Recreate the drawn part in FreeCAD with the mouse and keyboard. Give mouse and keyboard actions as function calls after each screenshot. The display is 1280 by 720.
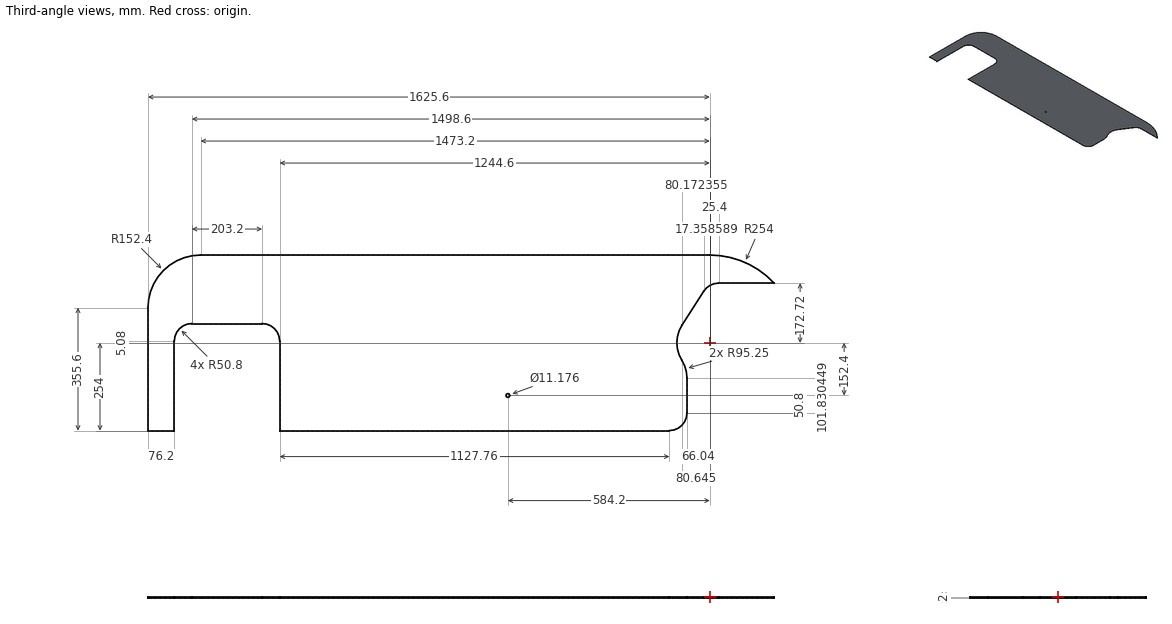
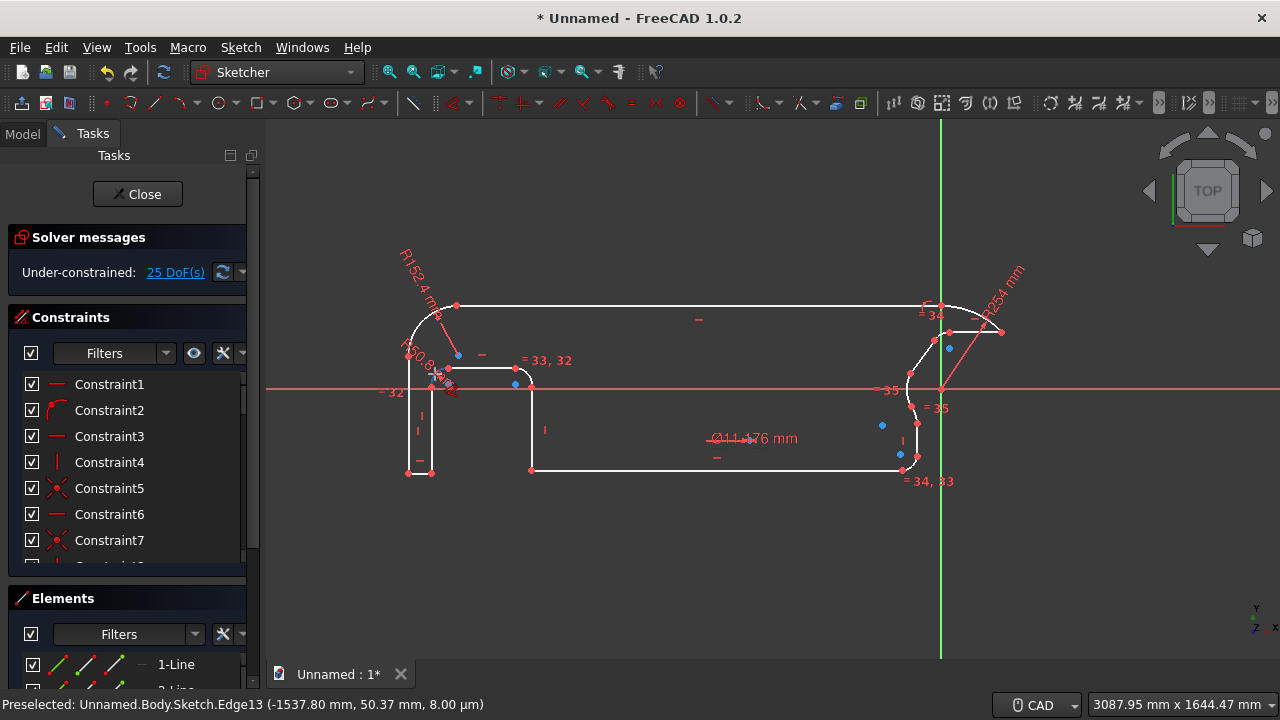
scroll(916, 418, up, 5)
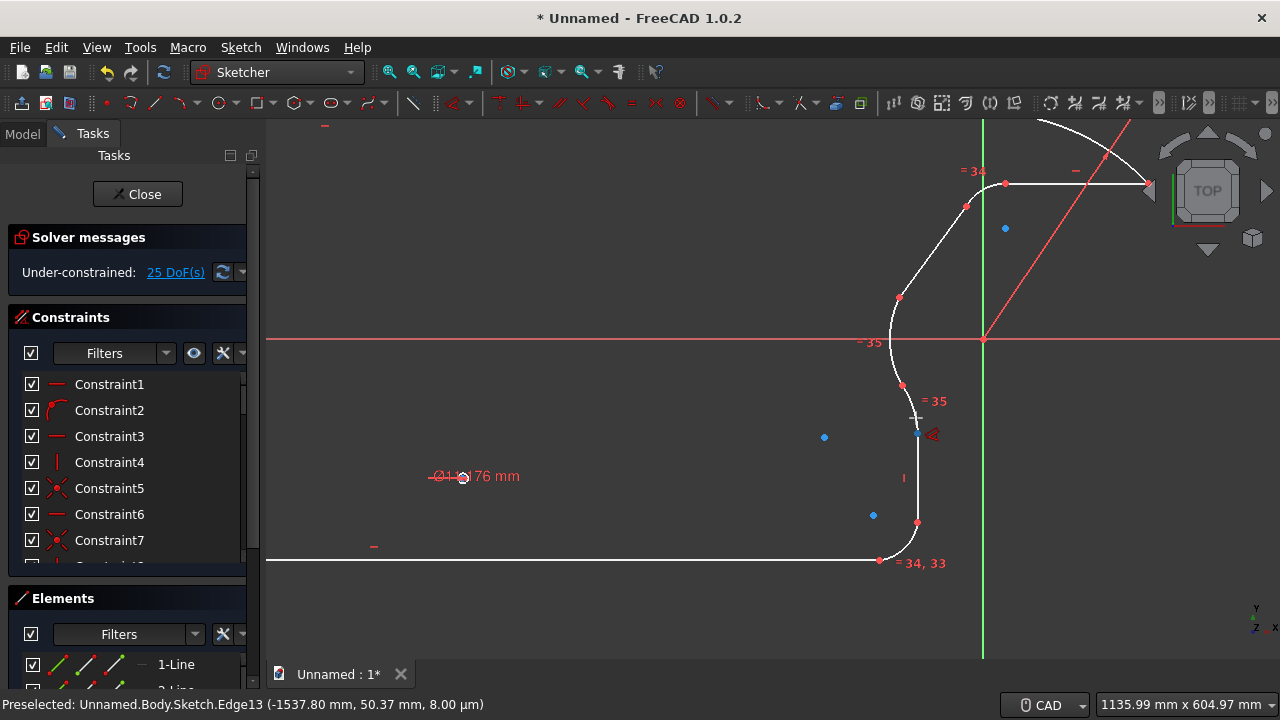
click(916, 418)
click(947, 411)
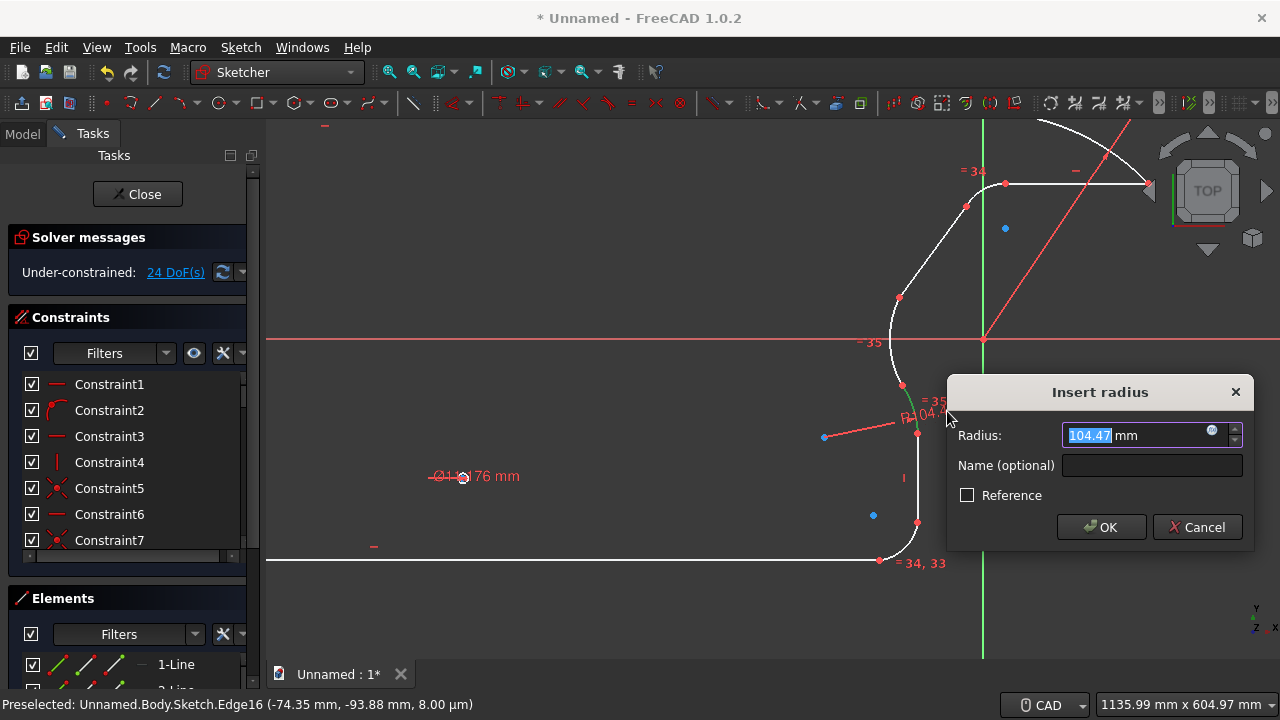
text(95.25)
key(Return)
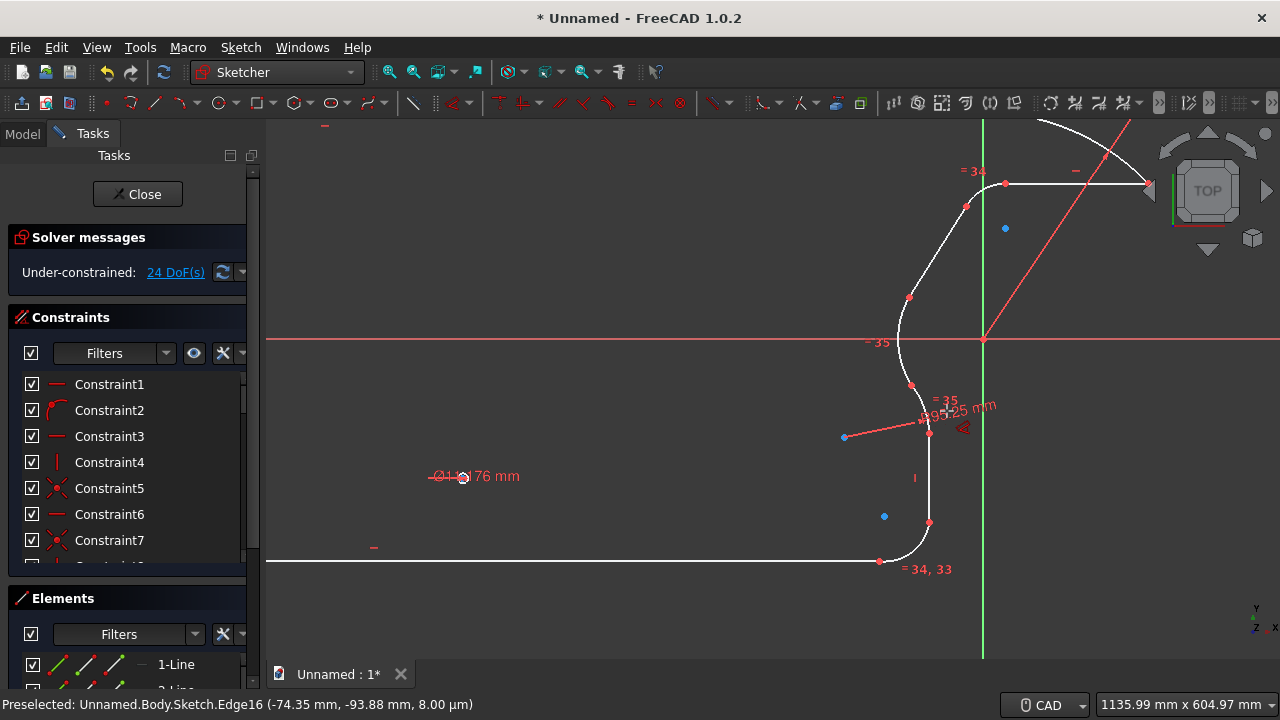
scroll(916, 418, down, 5)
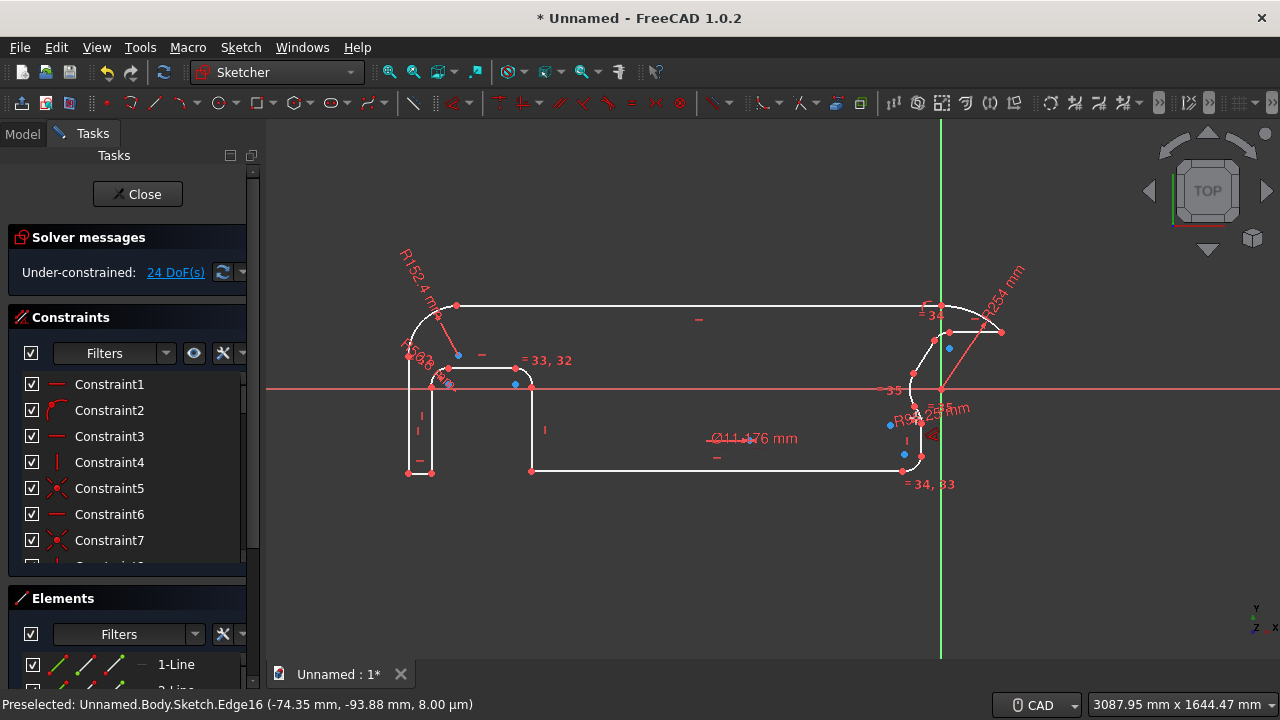
scroll(415, 474, up, 4)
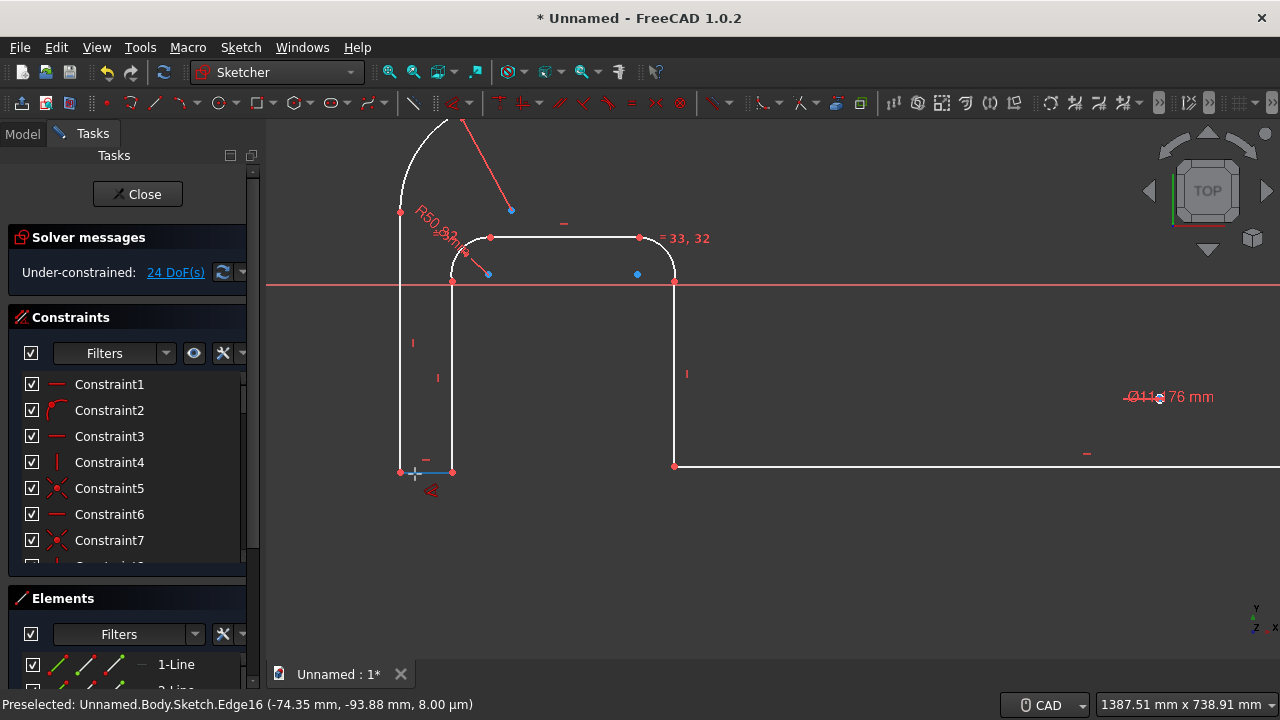
click(416, 473)
click(426, 507)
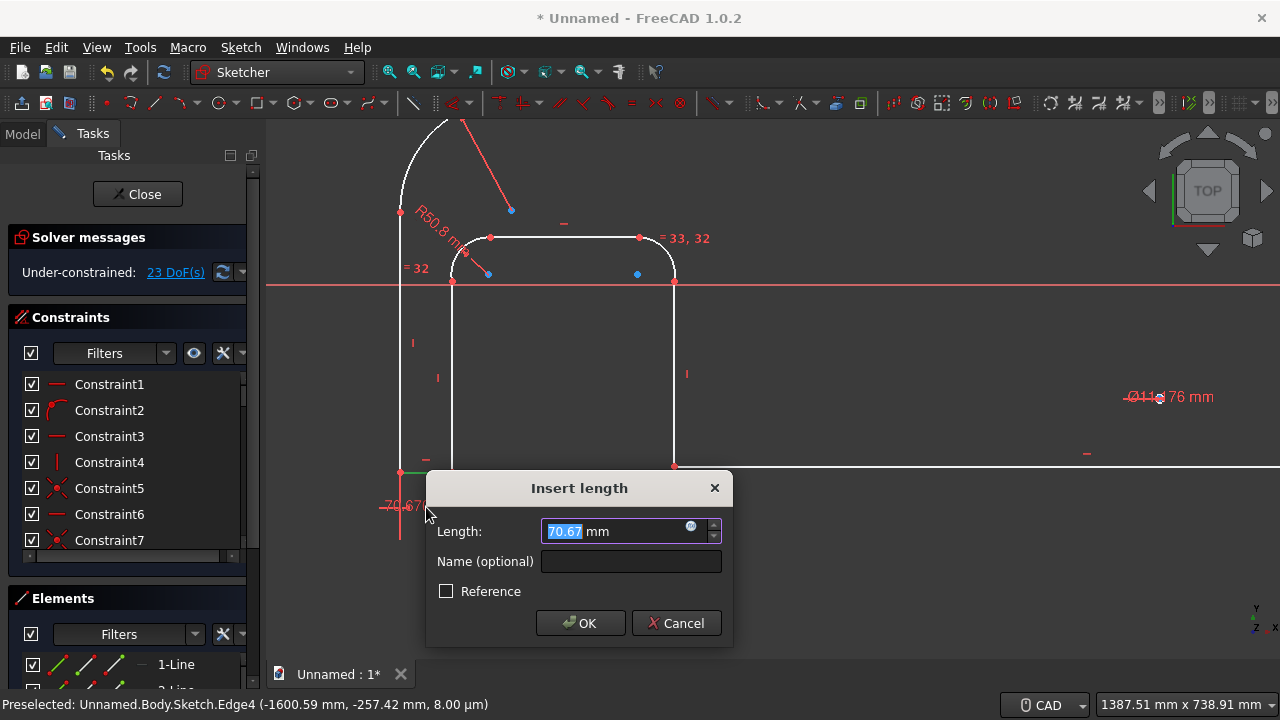
text(76.2)
key(Return)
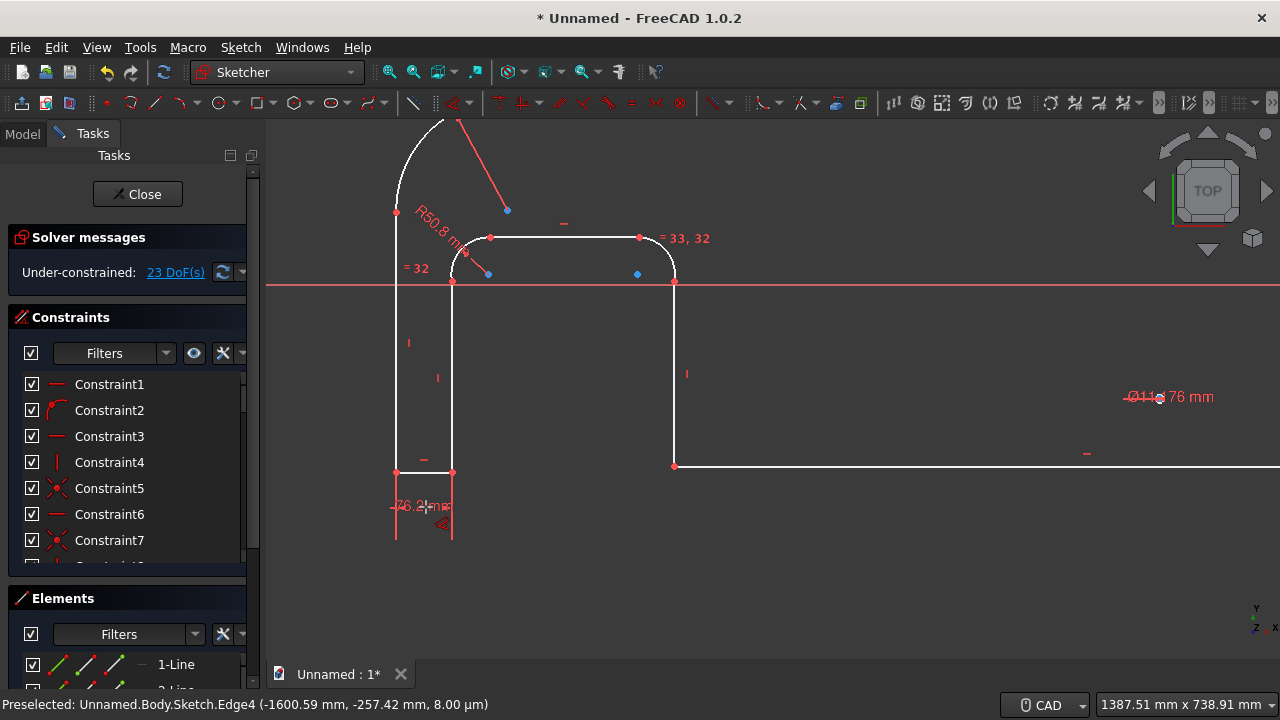
click(396, 473)
click(362, 379)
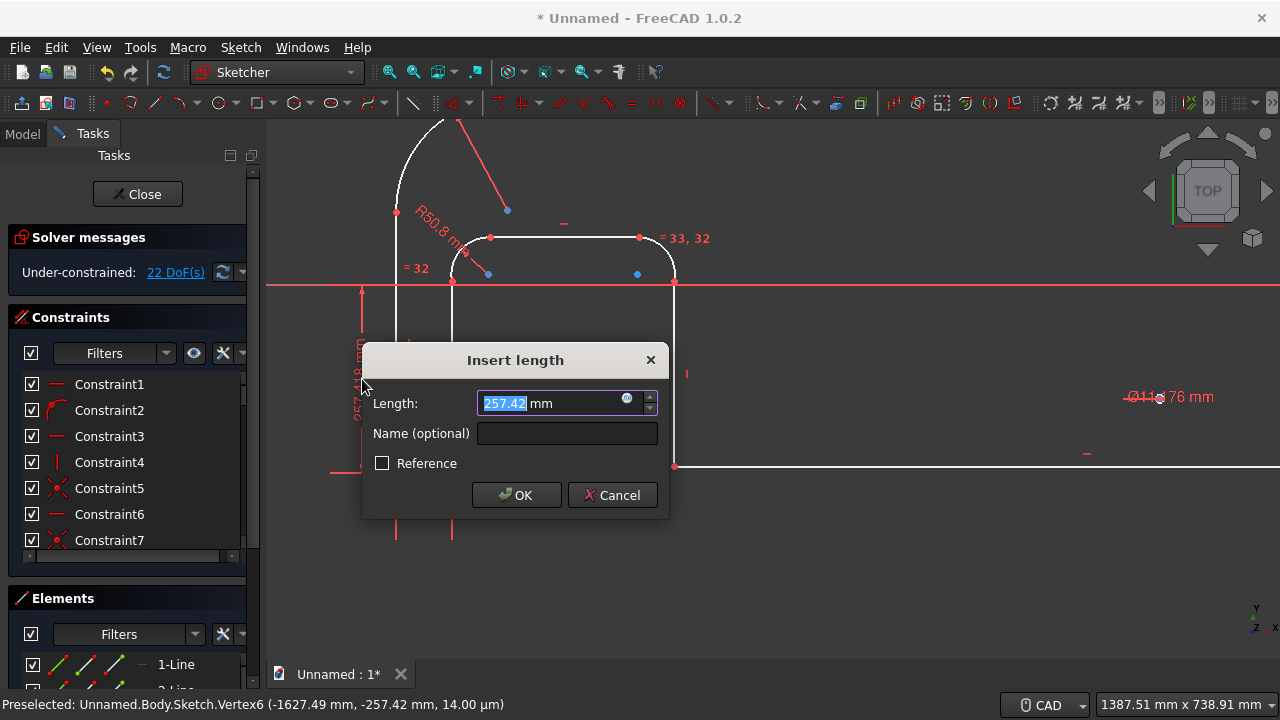
text(254)
key(Return)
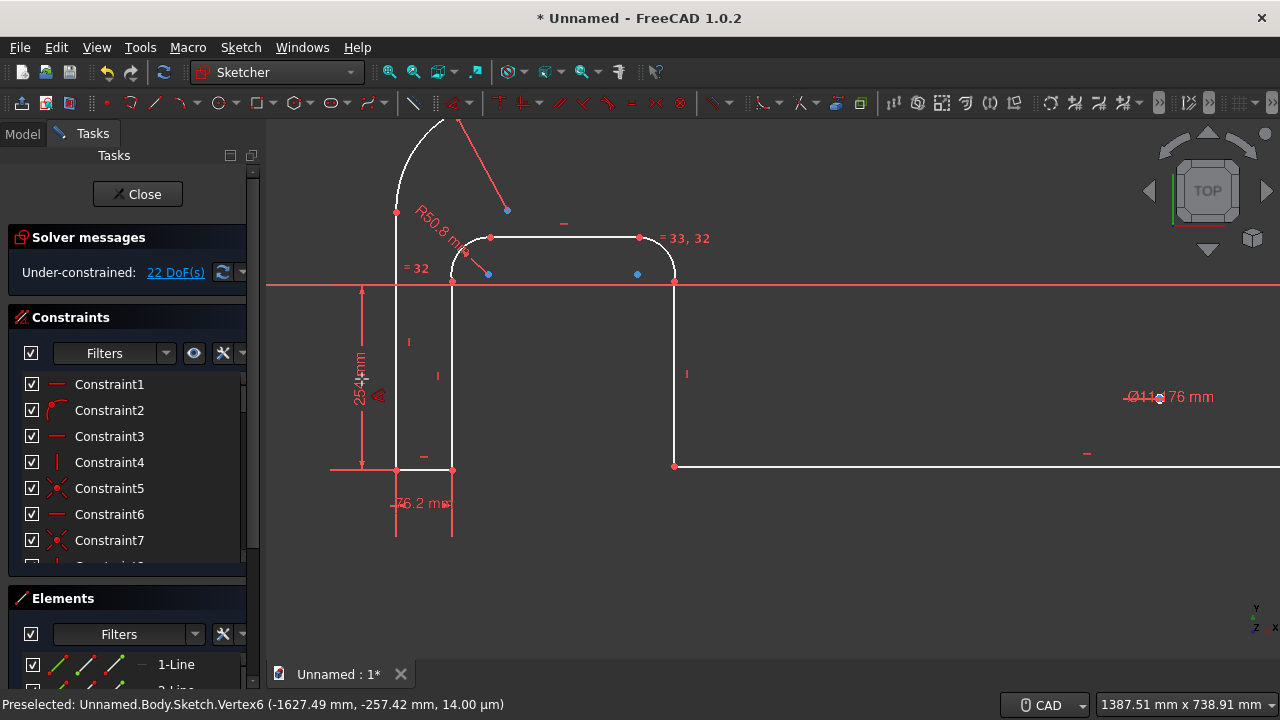
click(674, 467)
click(640, 376)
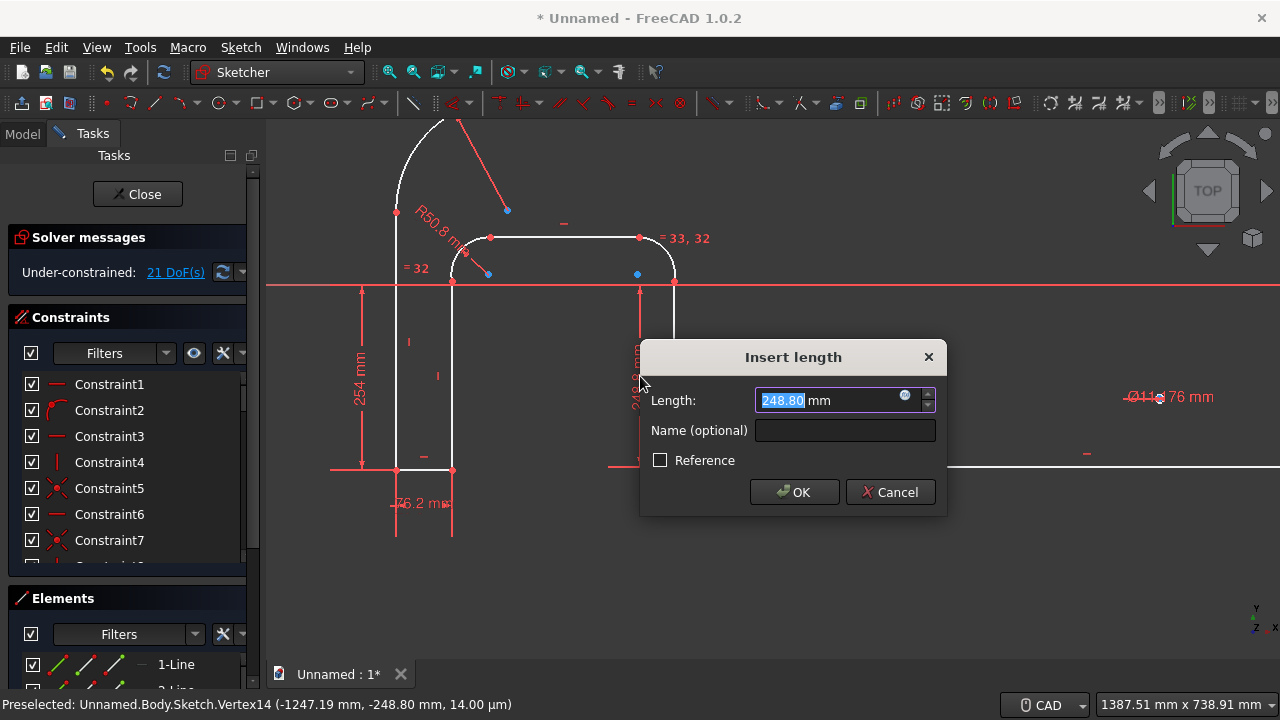
text(254)
key(Return)